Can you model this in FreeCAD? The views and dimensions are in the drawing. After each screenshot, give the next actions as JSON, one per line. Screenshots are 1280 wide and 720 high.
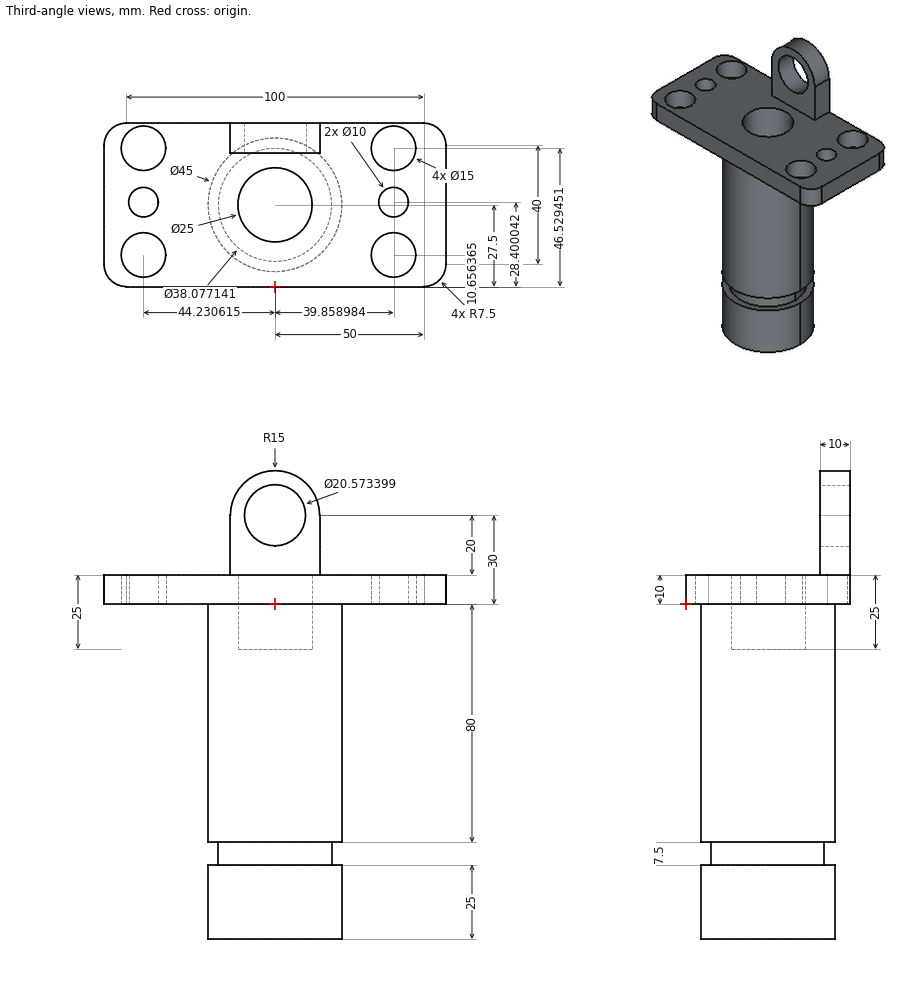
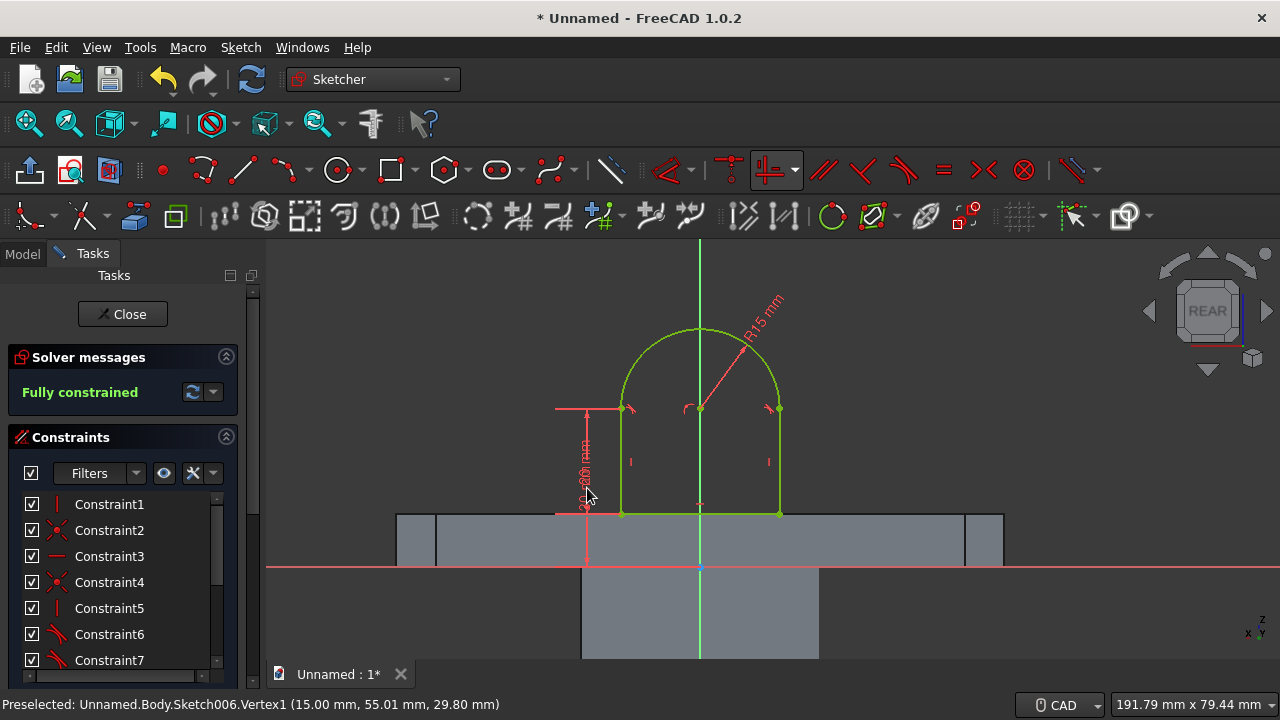
{"action": "left_click", "coordinate": [123, 314]}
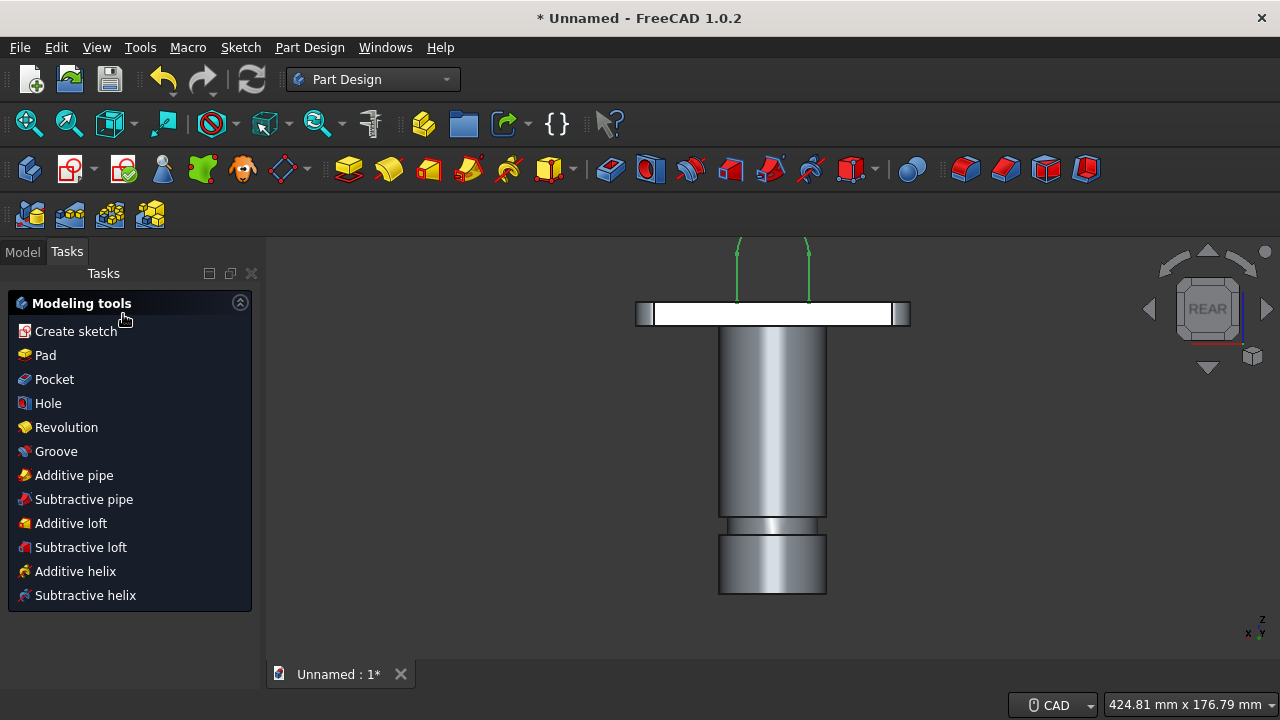
{"action": "left_click", "coordinate": [350, 170]}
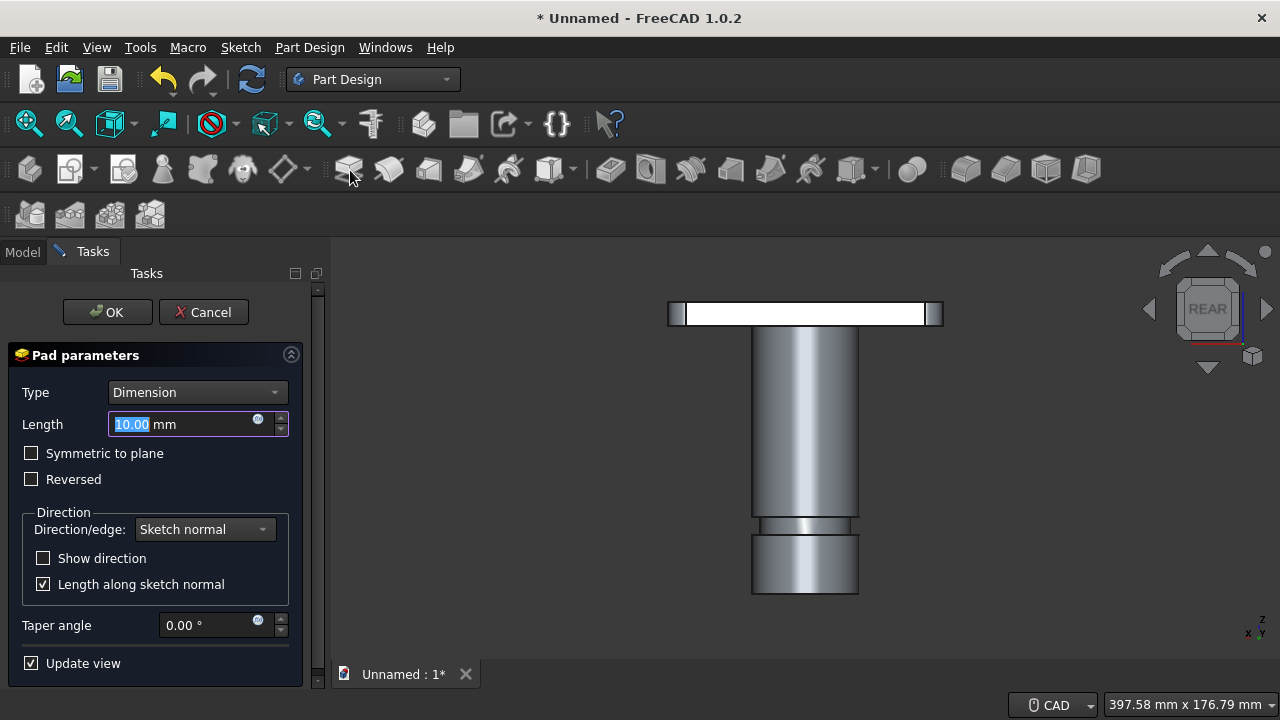
{"action": "type", "text": "10"}
{"action": "key", "text": "Tab"}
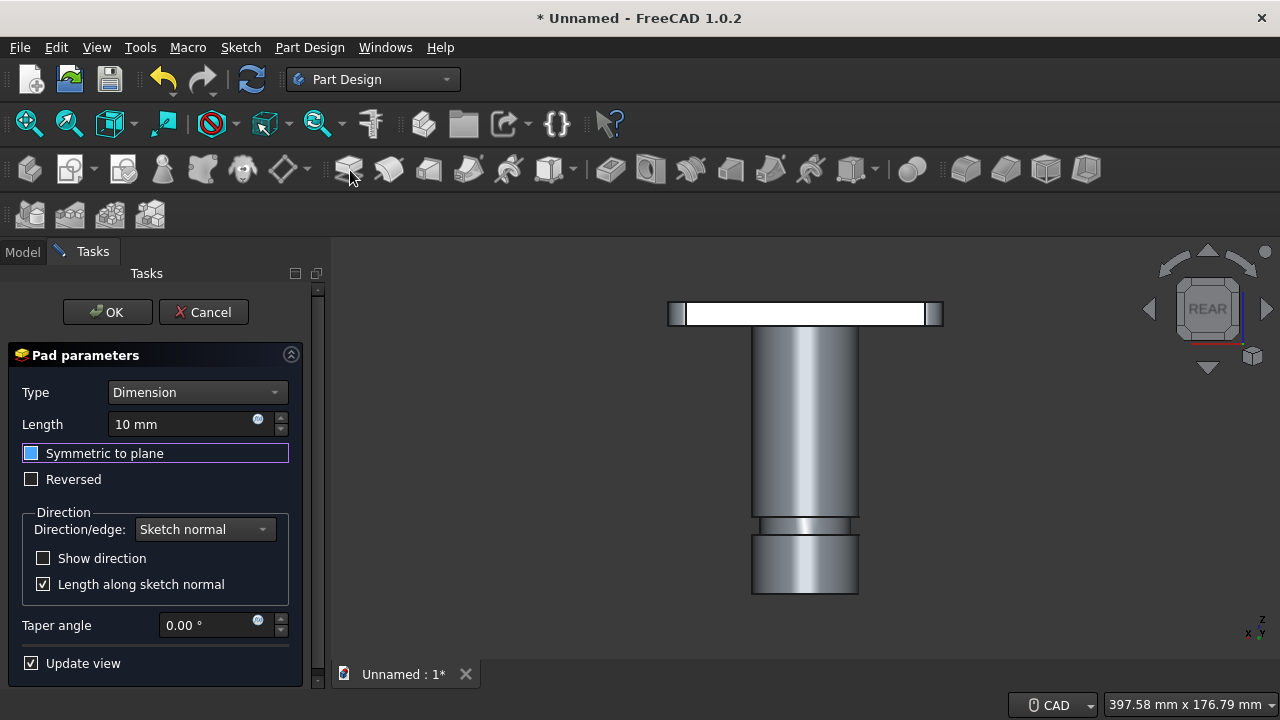
{"action": "left_click", "coordinate": [30, 479]}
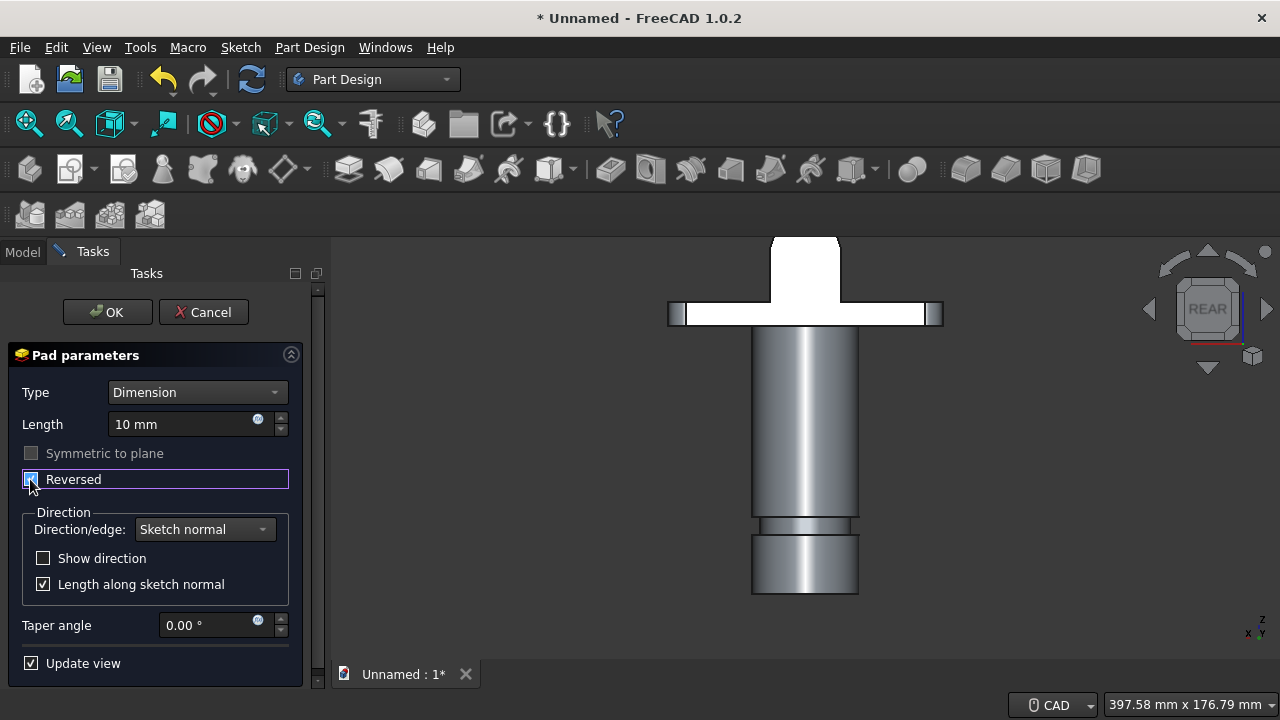
{"action": "left_click", "coordinate": [108, 312]}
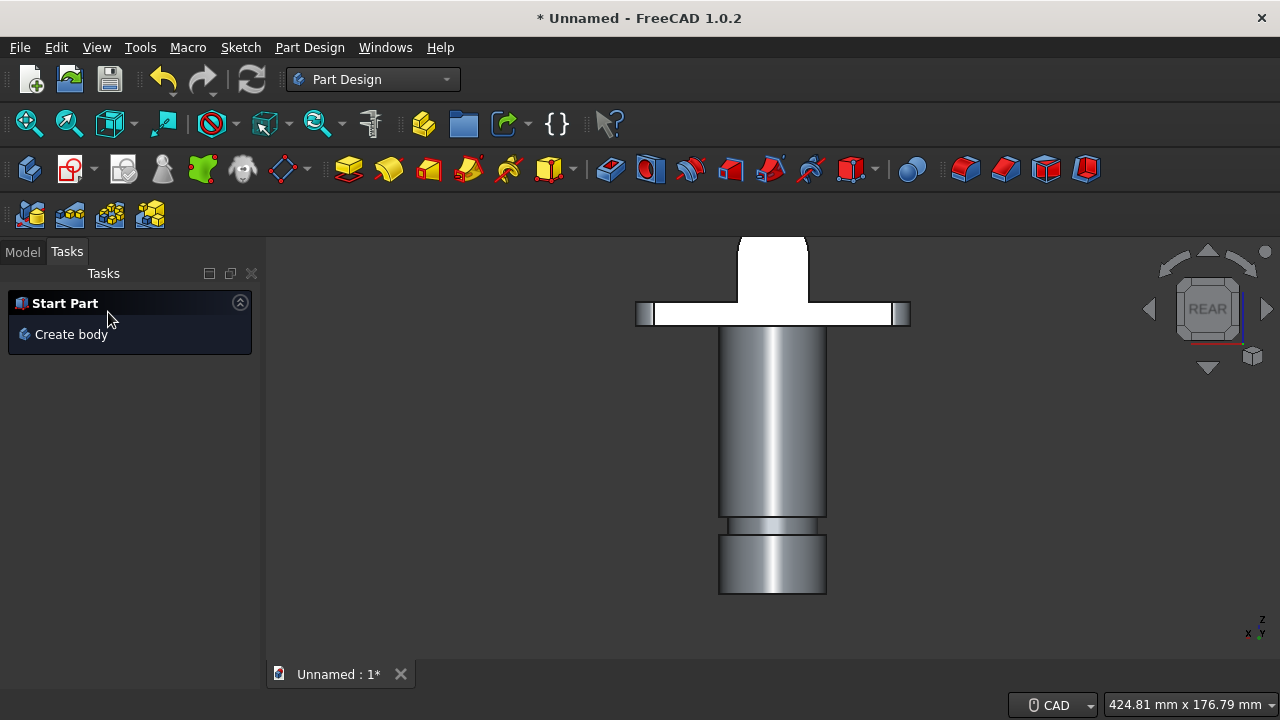
{"action": "left_click", "coordinate": [30, 124]}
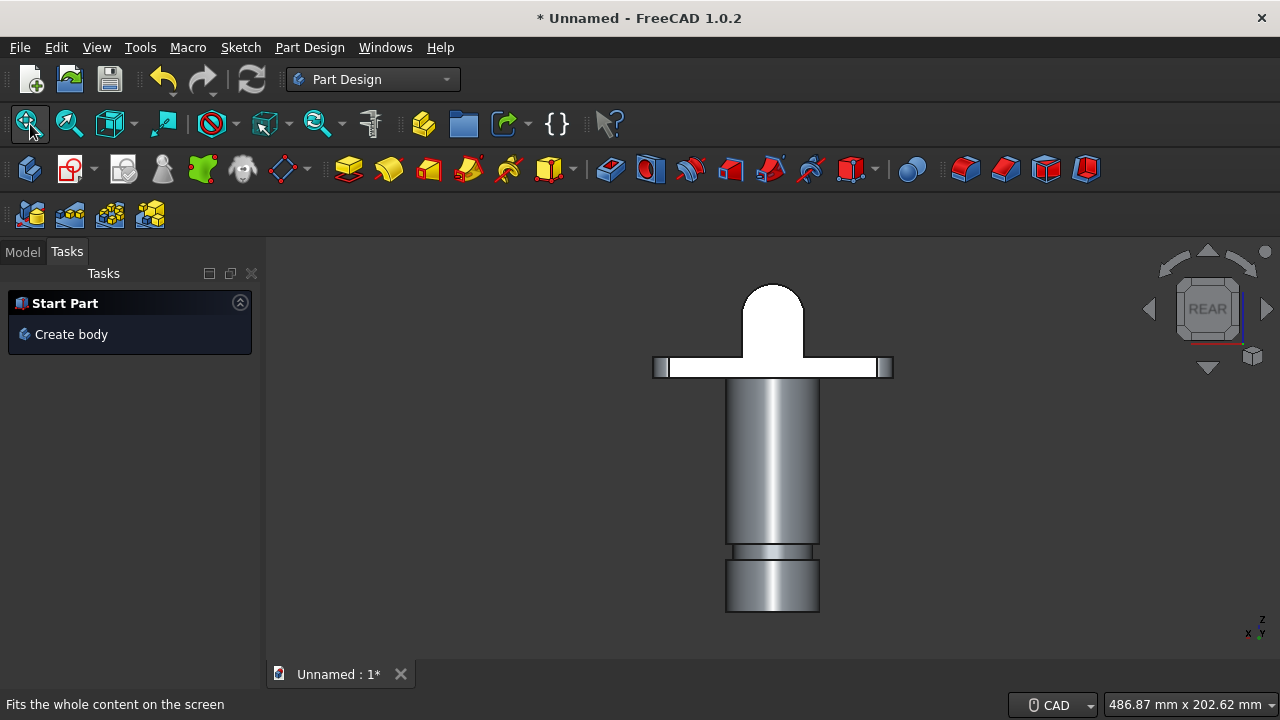
{"action": "key", "text": "0"}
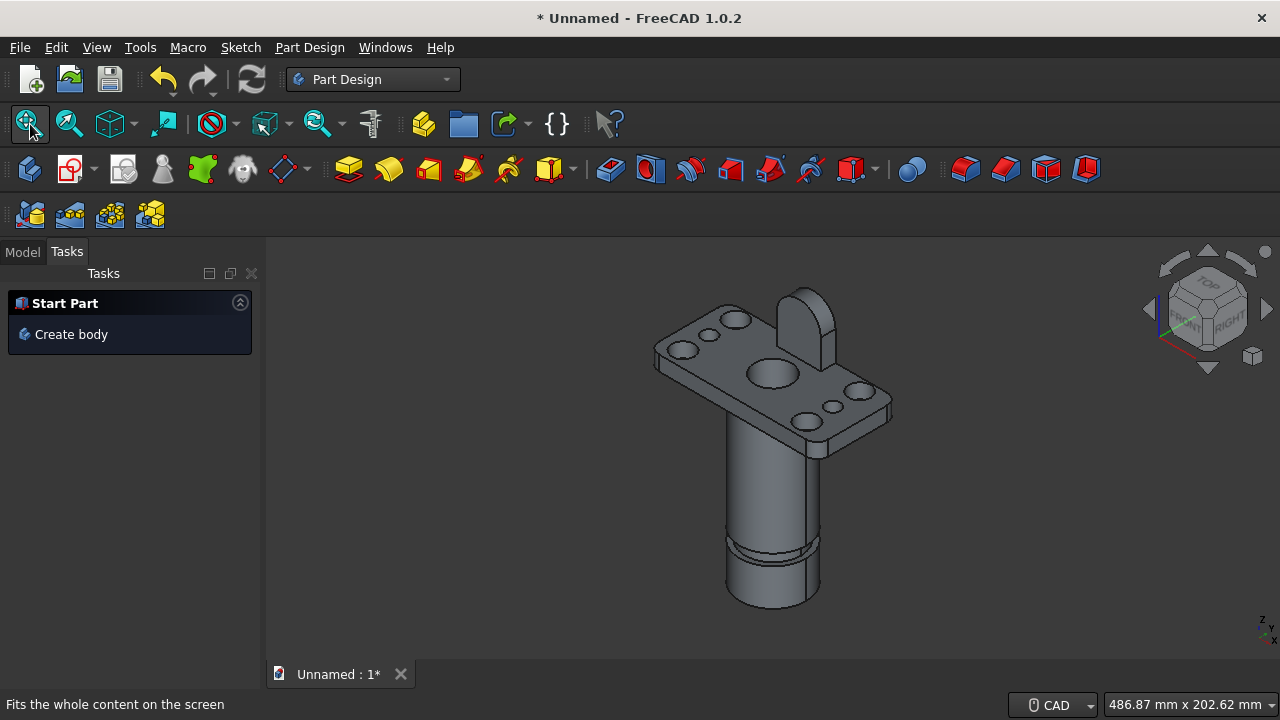
{"action": "left_click", "coordinate": [799, 328]}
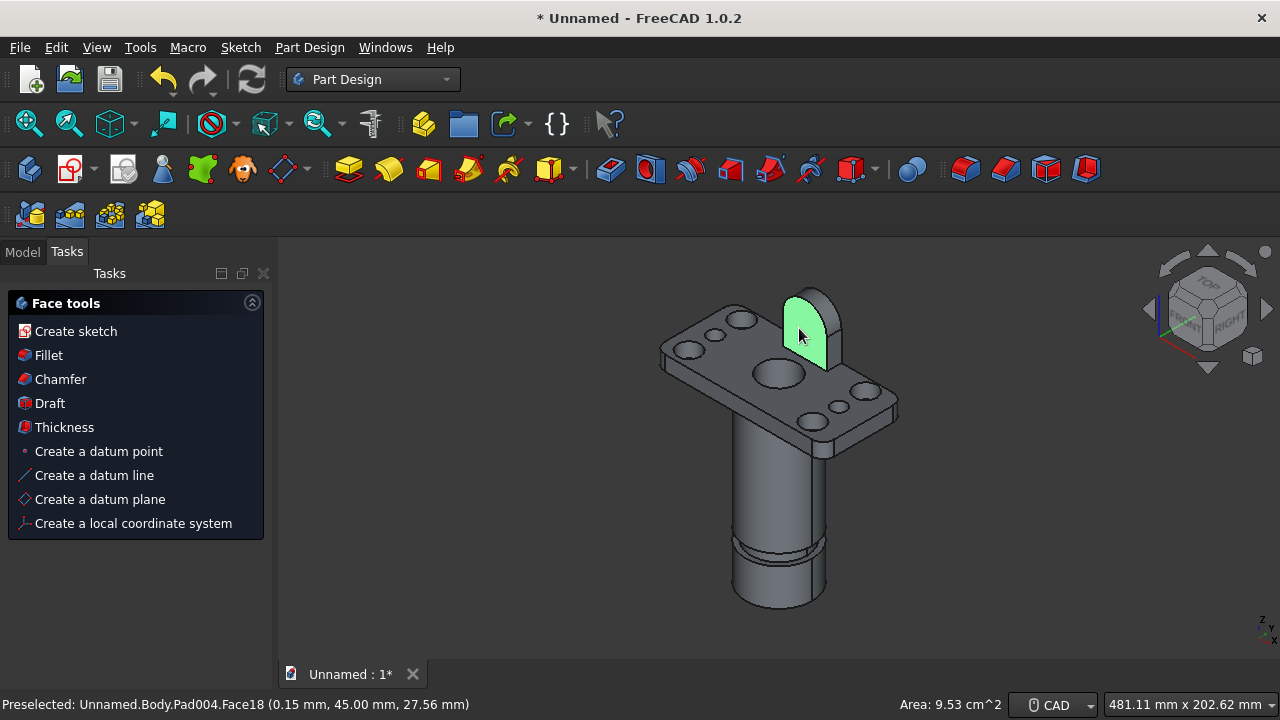
{"action": "left_click", "coordinate": [70, 170]}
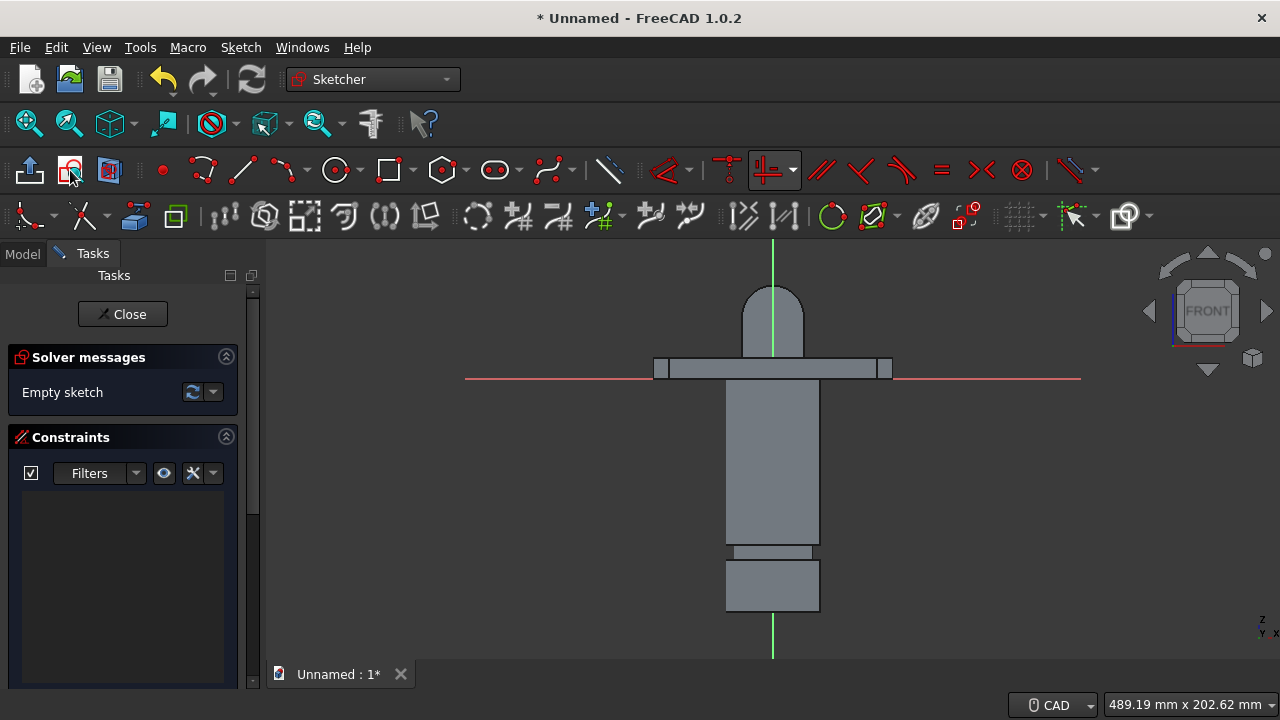
{"action": "scroll", "coordinate": [803, 289], "scroll_direction": "up", "scroll_amount": 6}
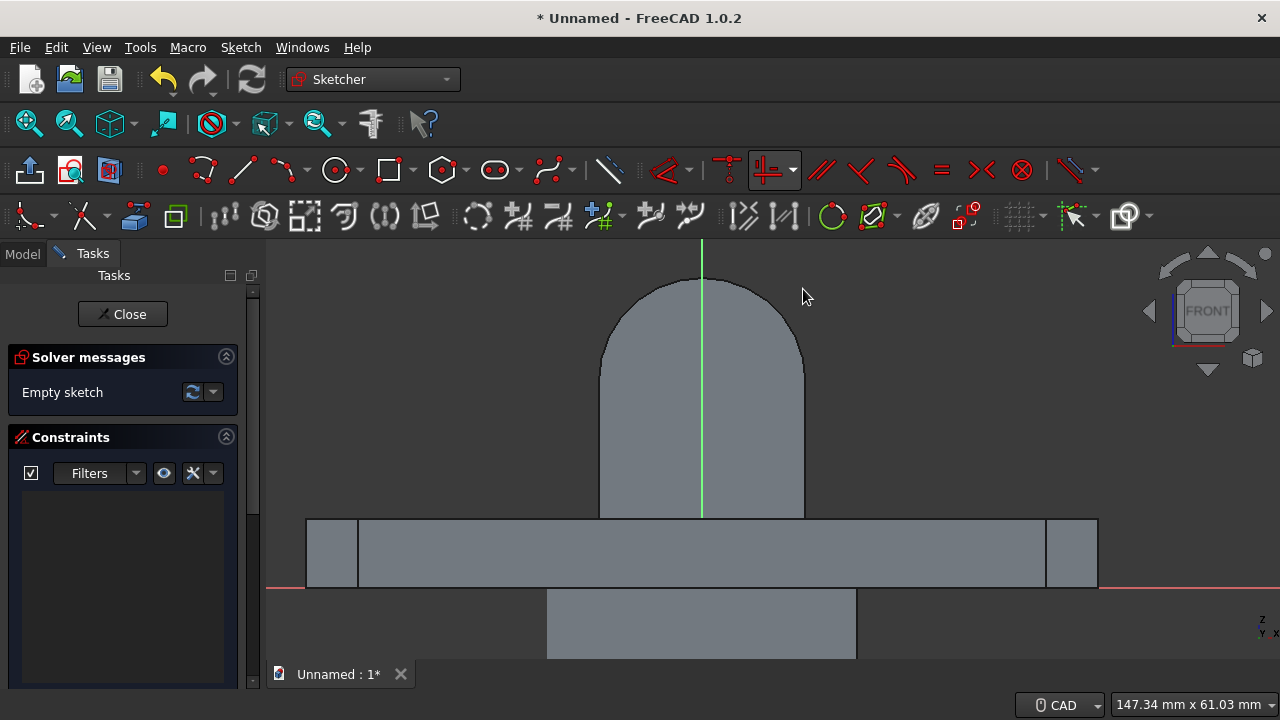
{"action": "key", "text": "g c"}